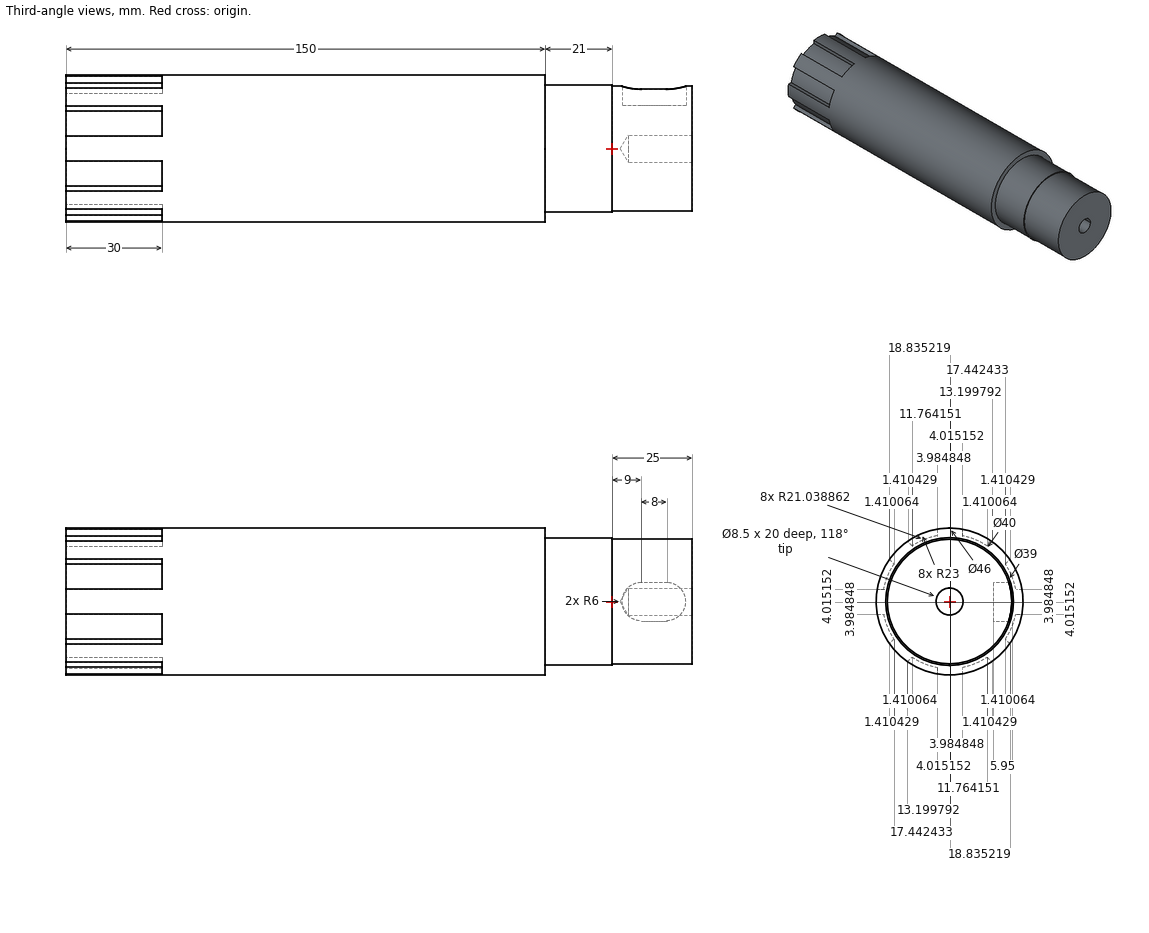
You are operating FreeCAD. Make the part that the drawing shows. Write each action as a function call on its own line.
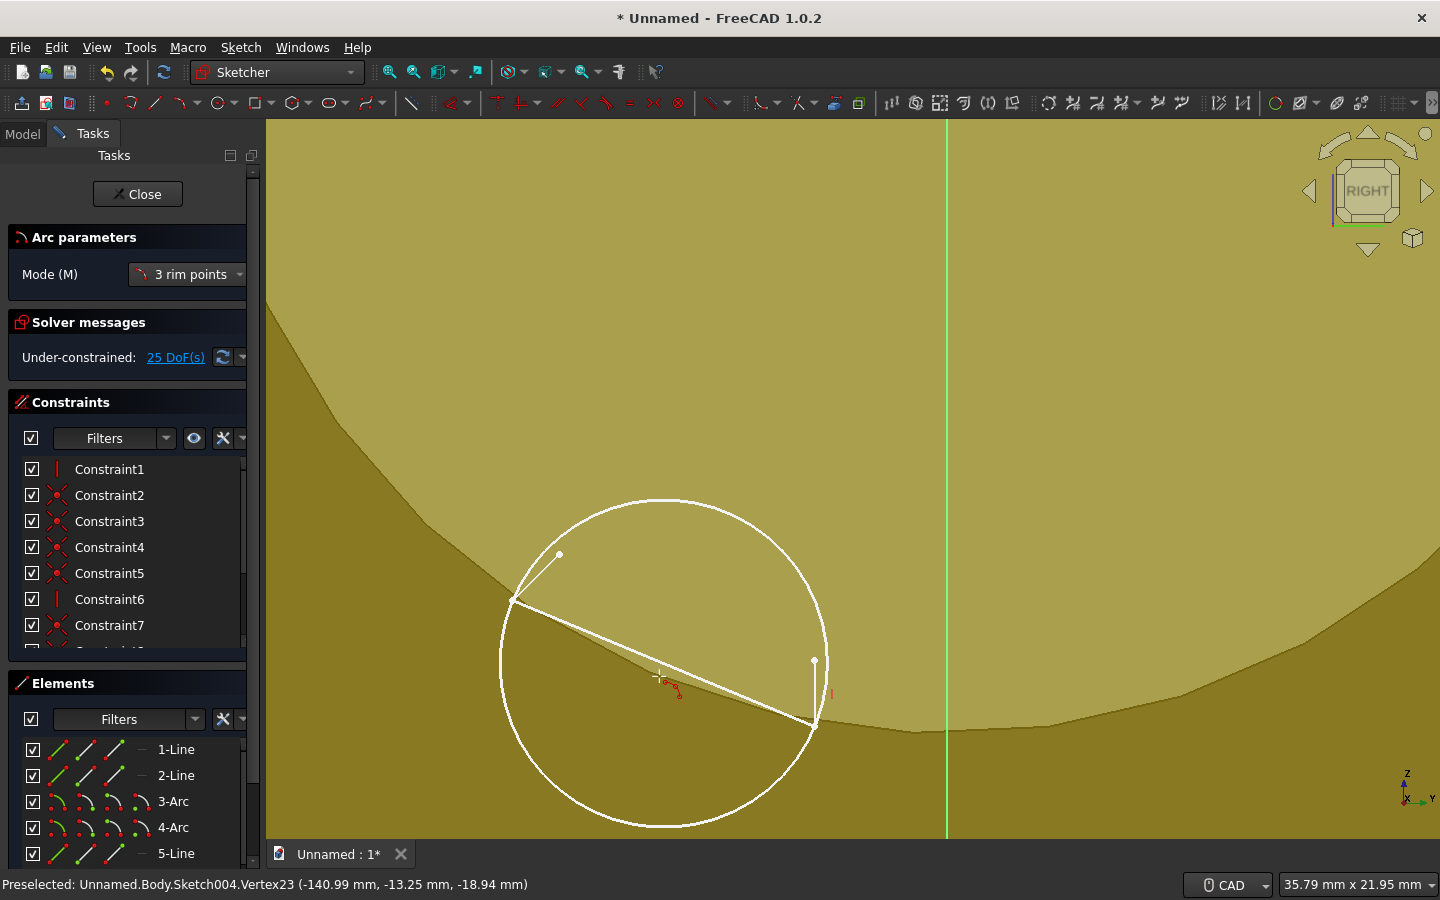
click(658, 676)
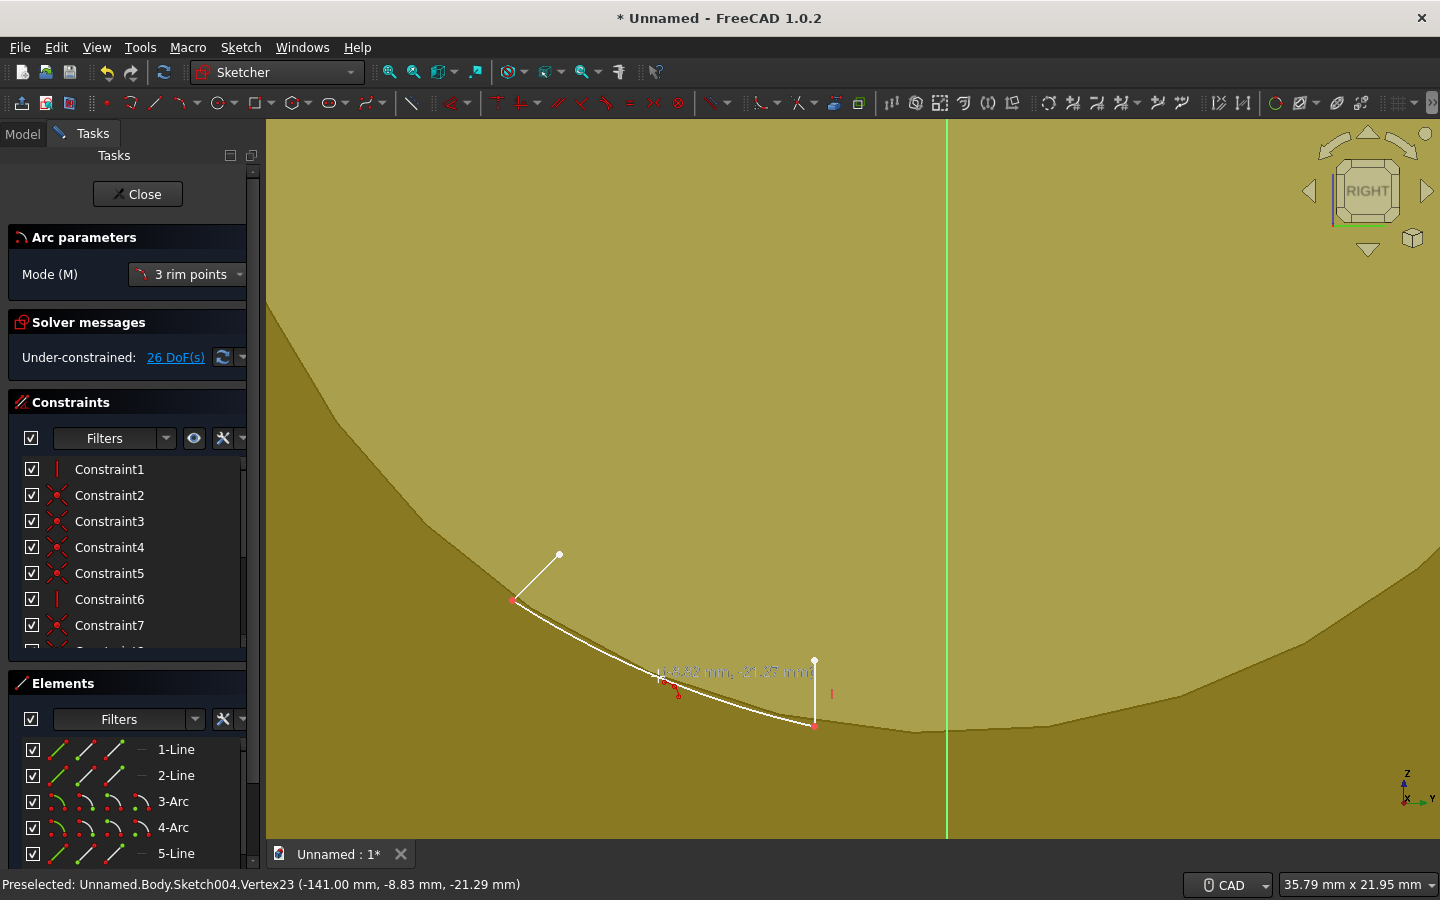
click(559, 554)
click(815, 660)
click(683, 617)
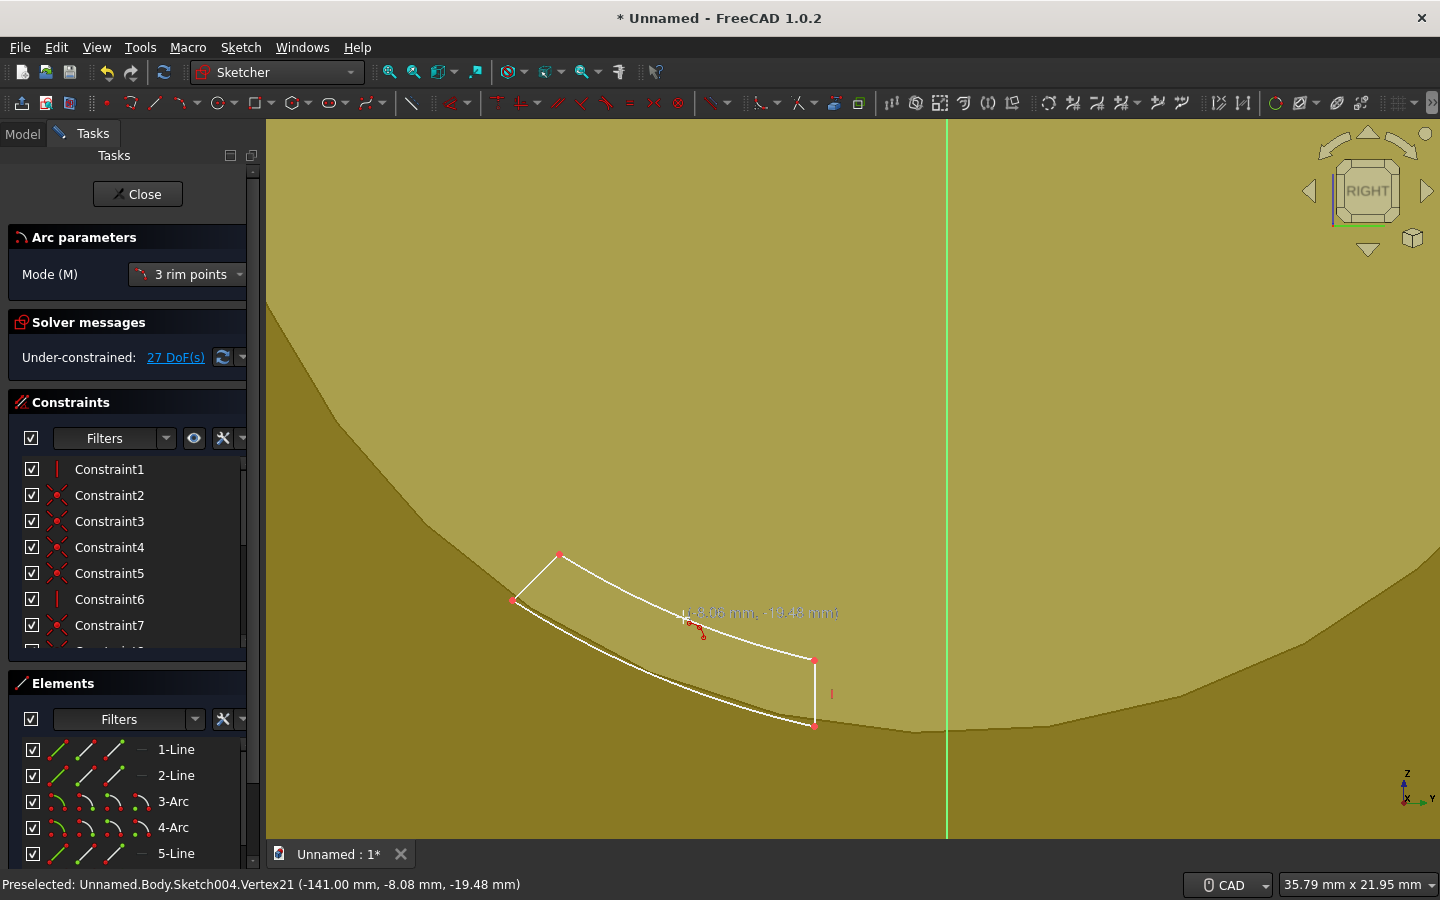
click(156, 104)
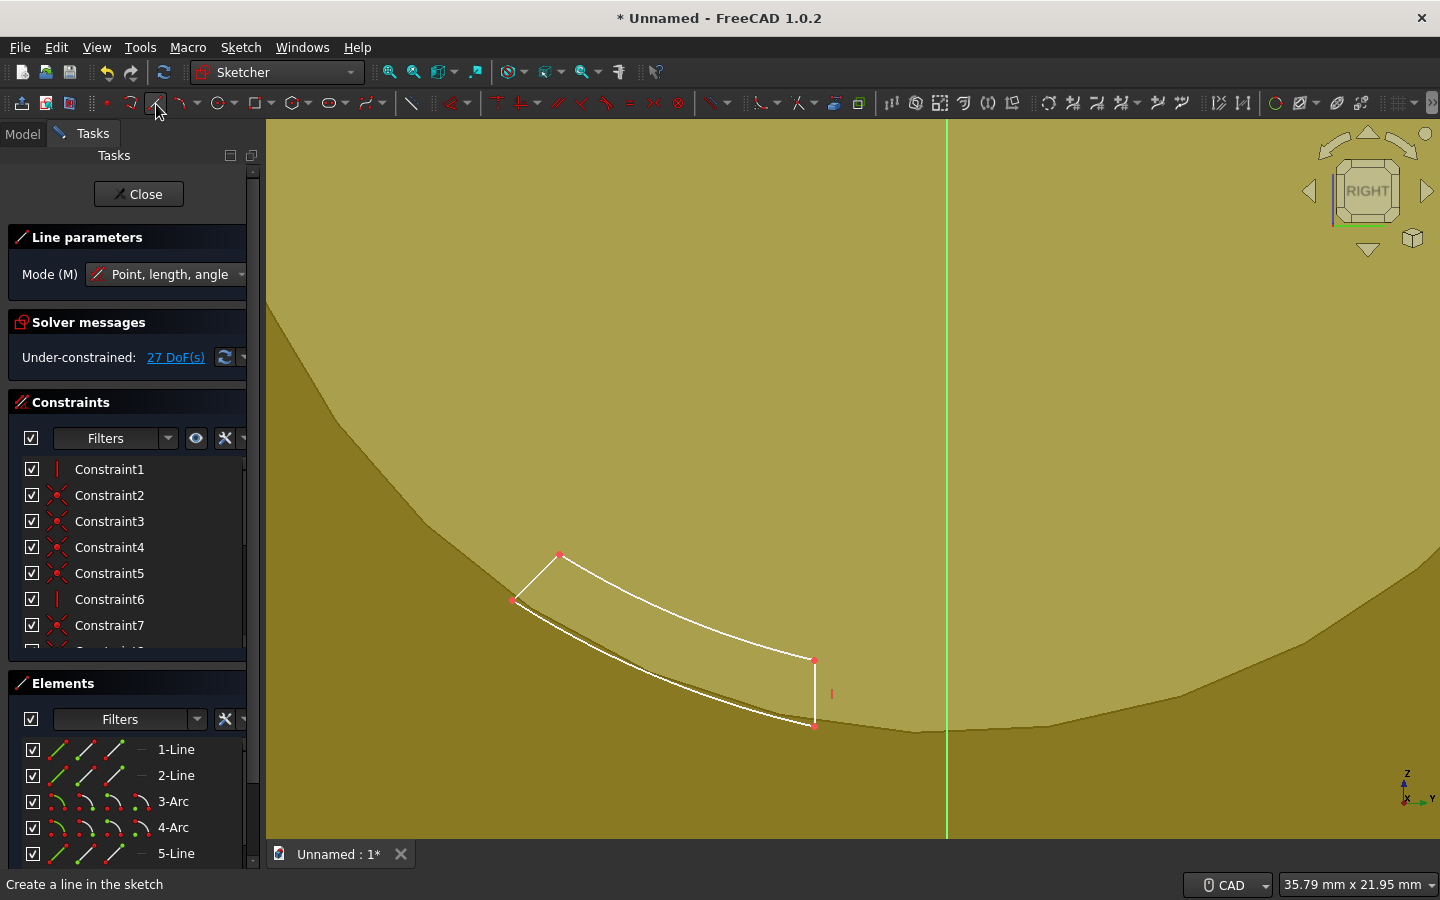
click(375, 365)
click(329, 411)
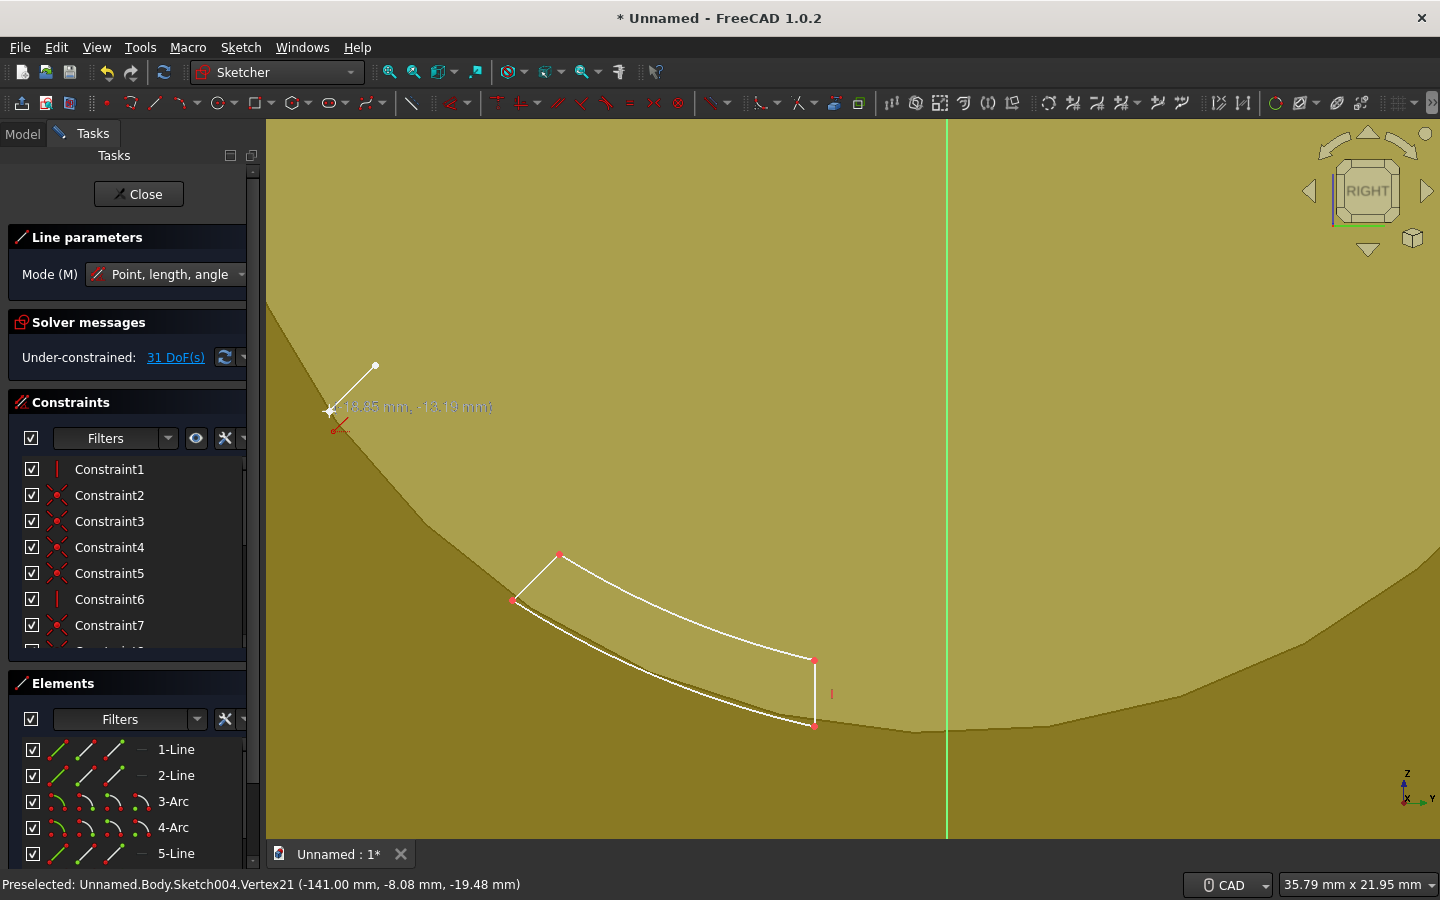
scroll(714, 694, down, 6)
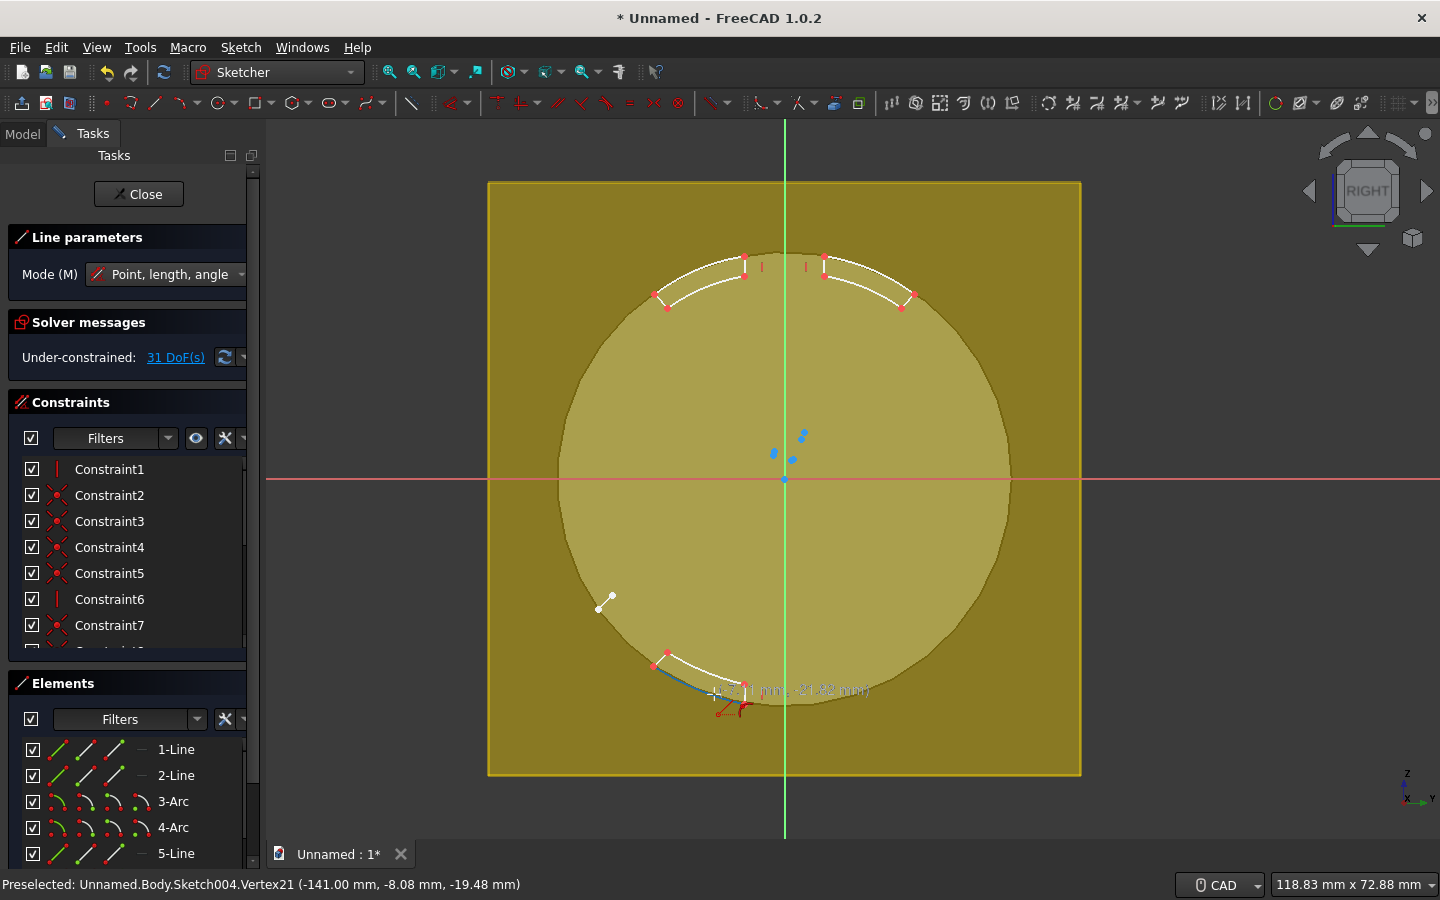
click(561, 519)
click(580, 519)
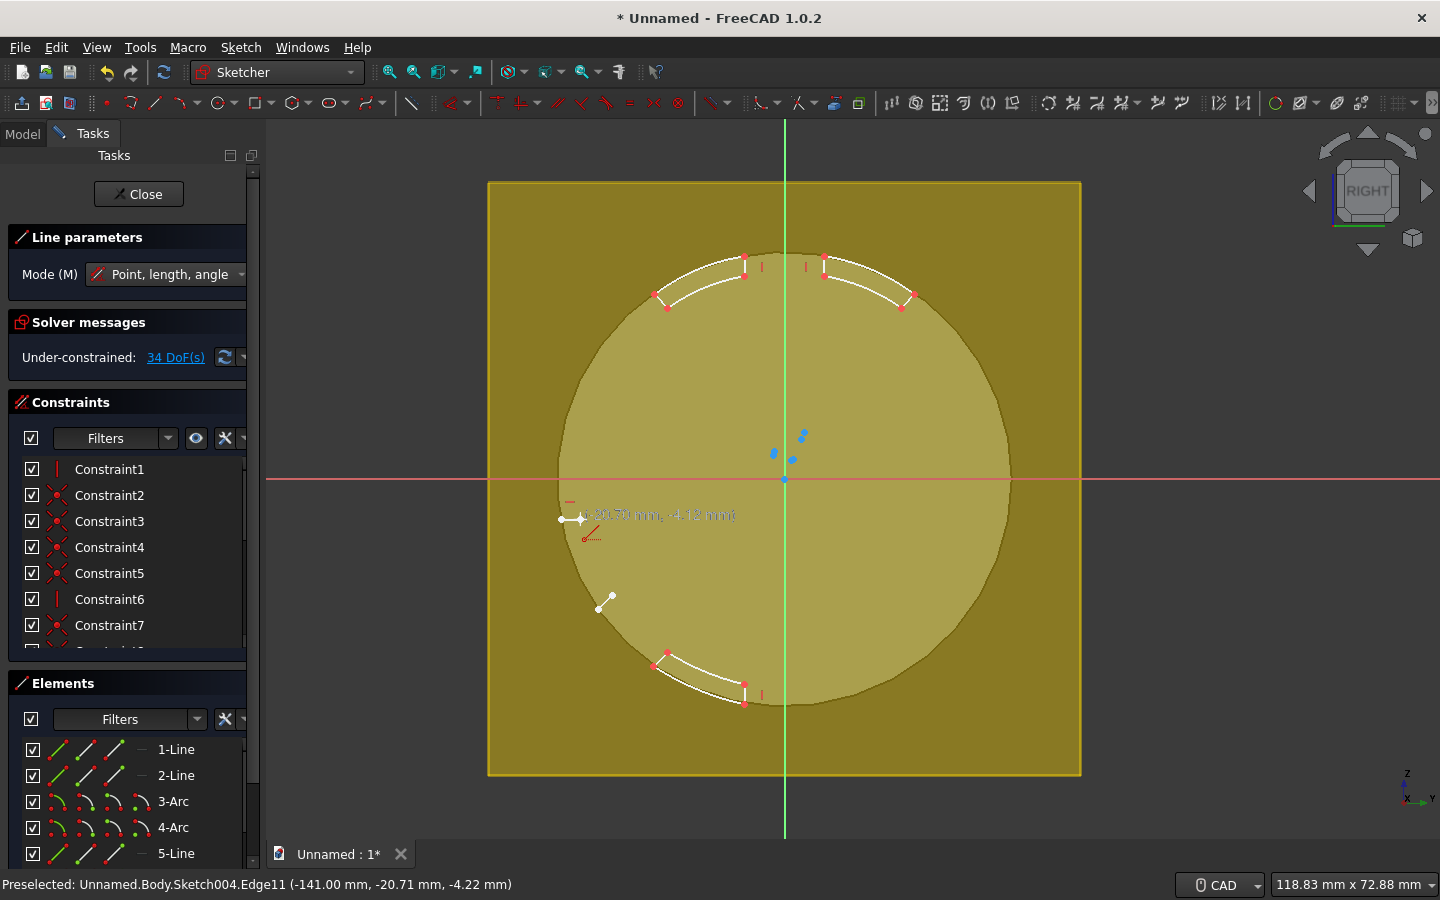
click(180, 104)